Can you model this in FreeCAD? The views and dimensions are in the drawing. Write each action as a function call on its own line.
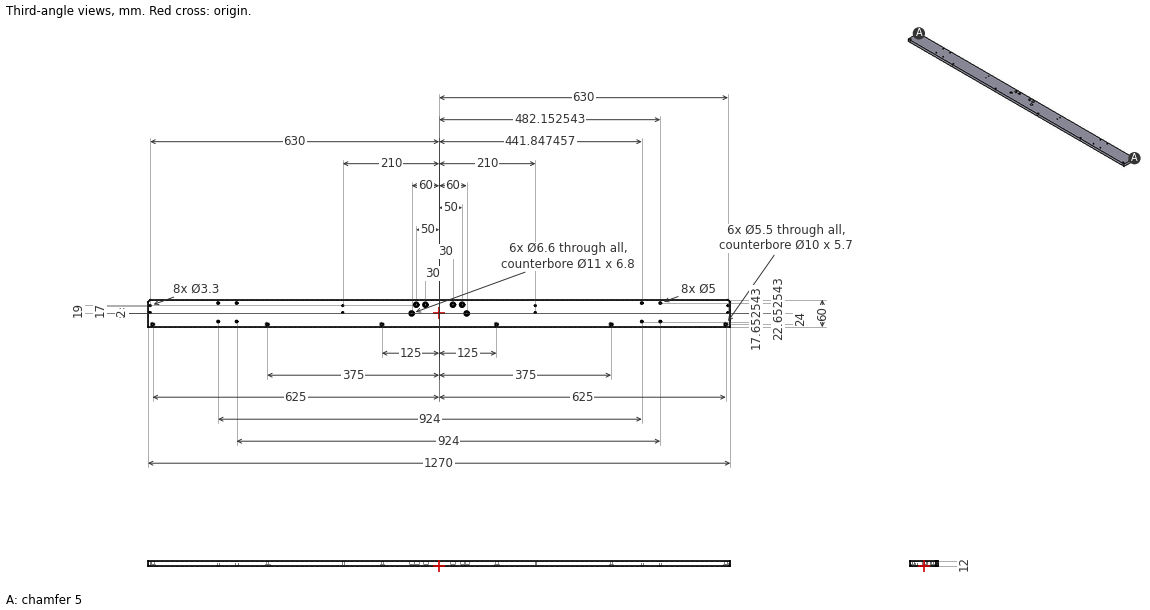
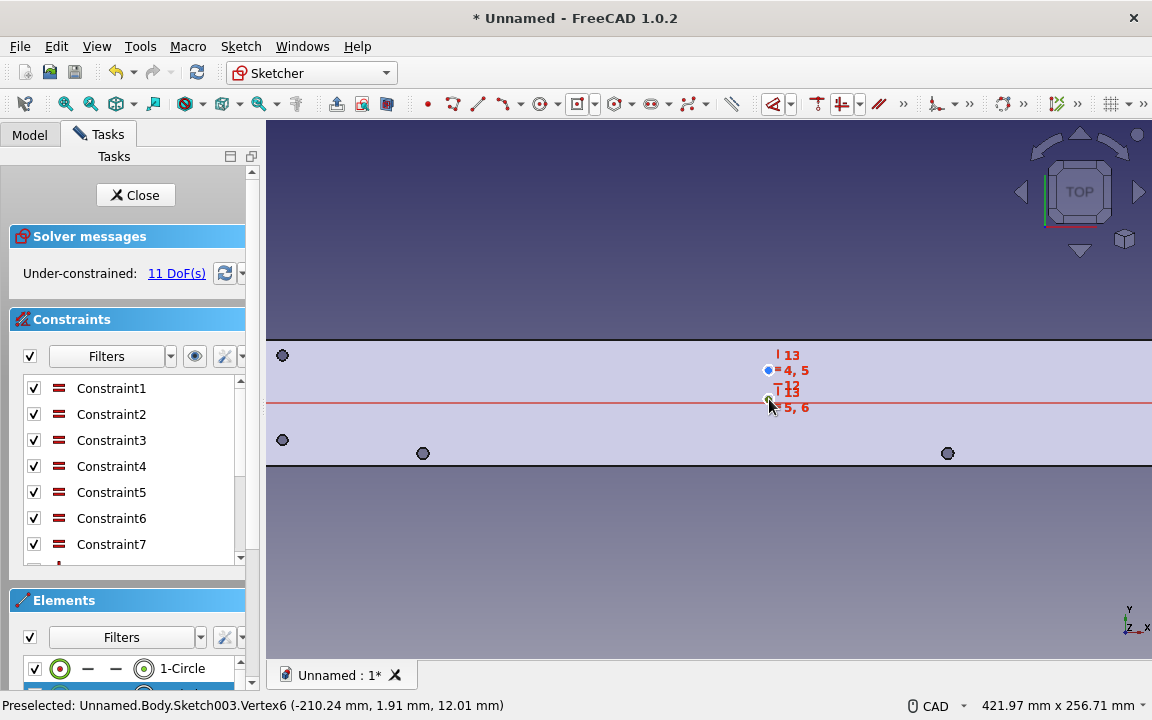
key(h)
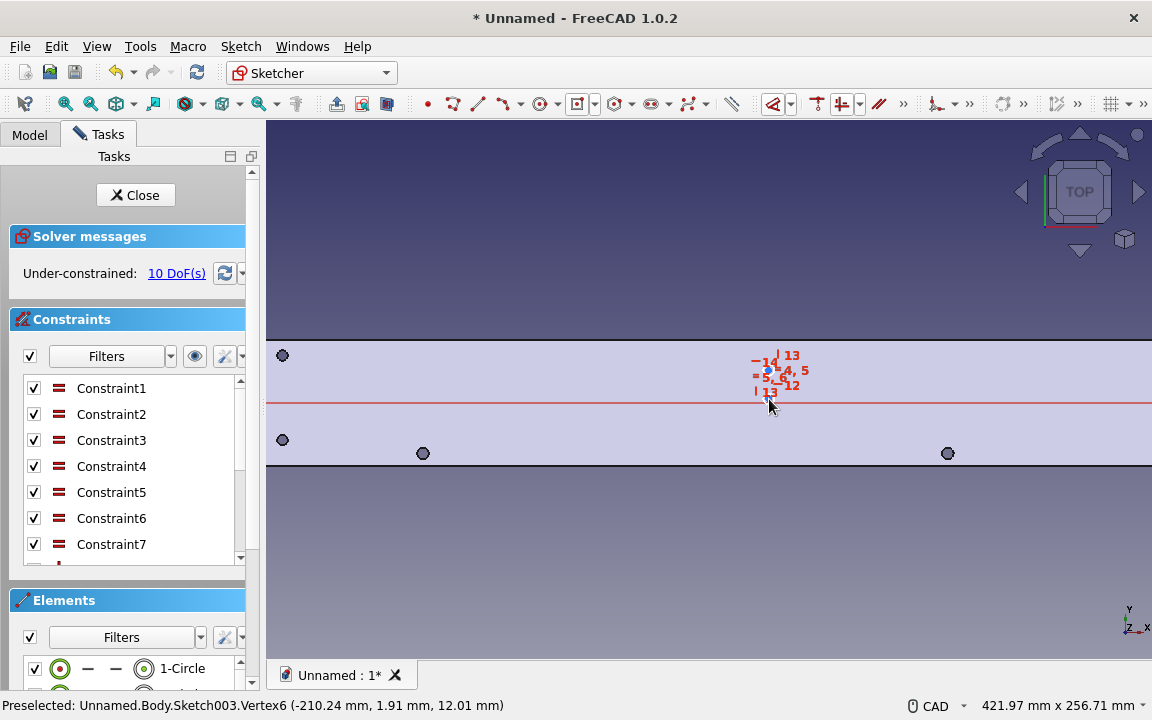
scroll(496, 391, down, 8)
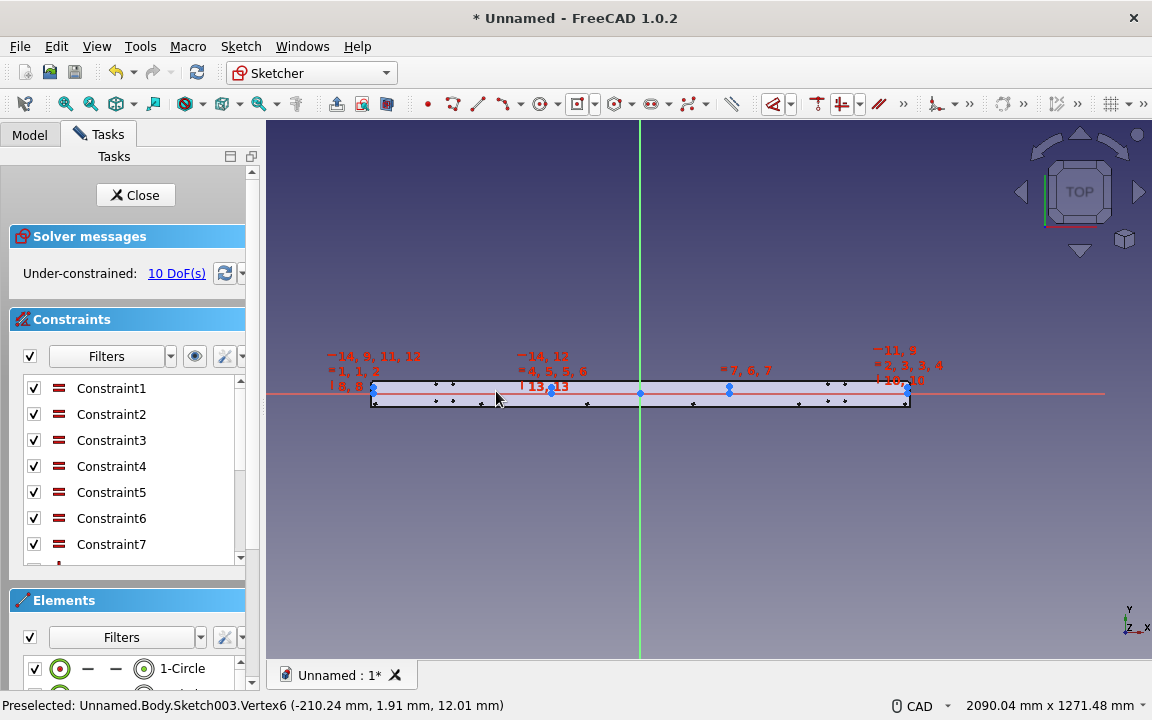
scroll(907, 393, up, 4)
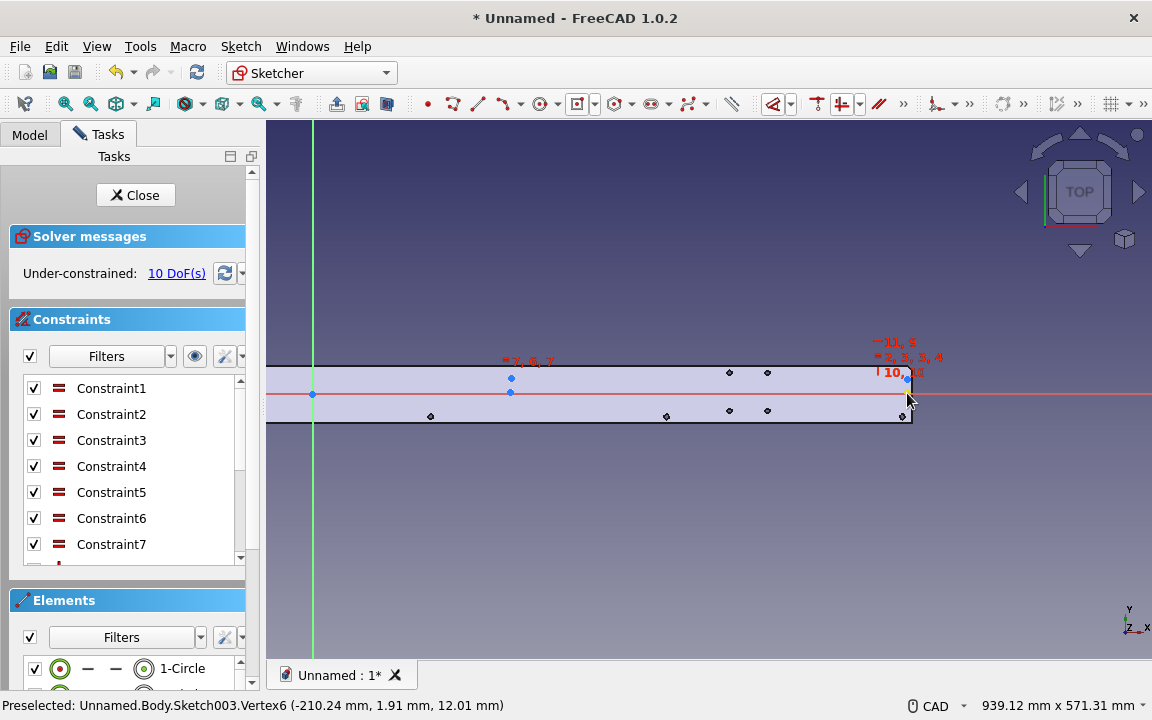
click(907, 392)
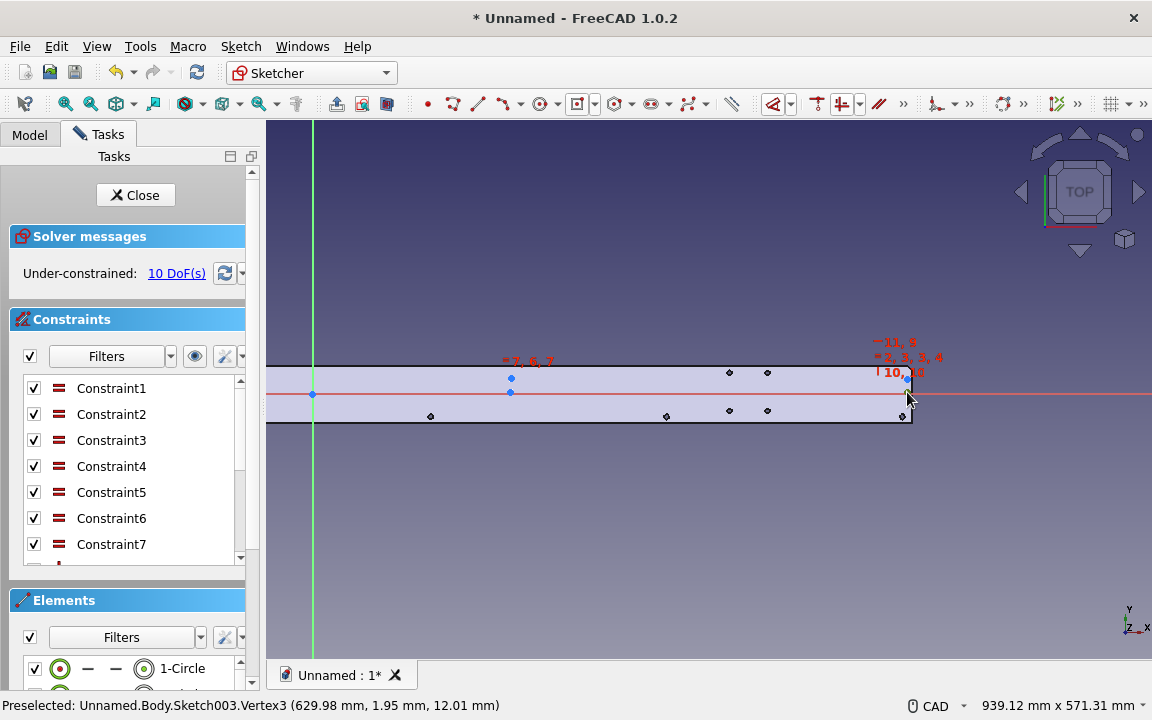
click(511, 392)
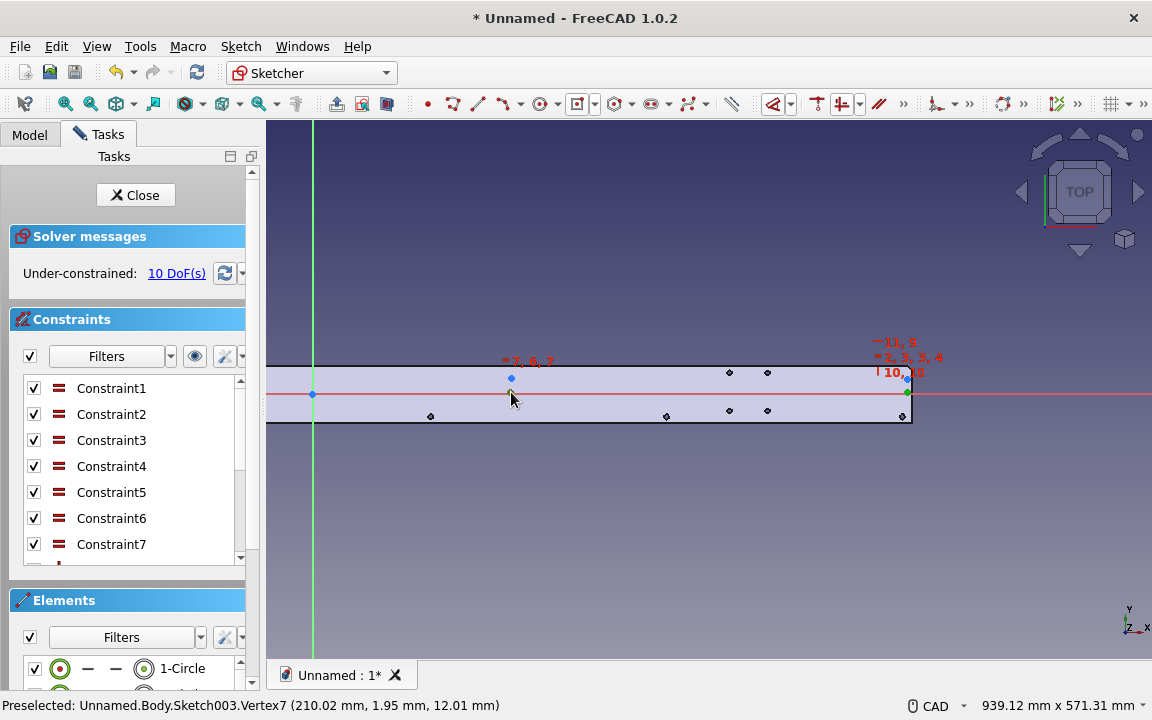
click(860, 104)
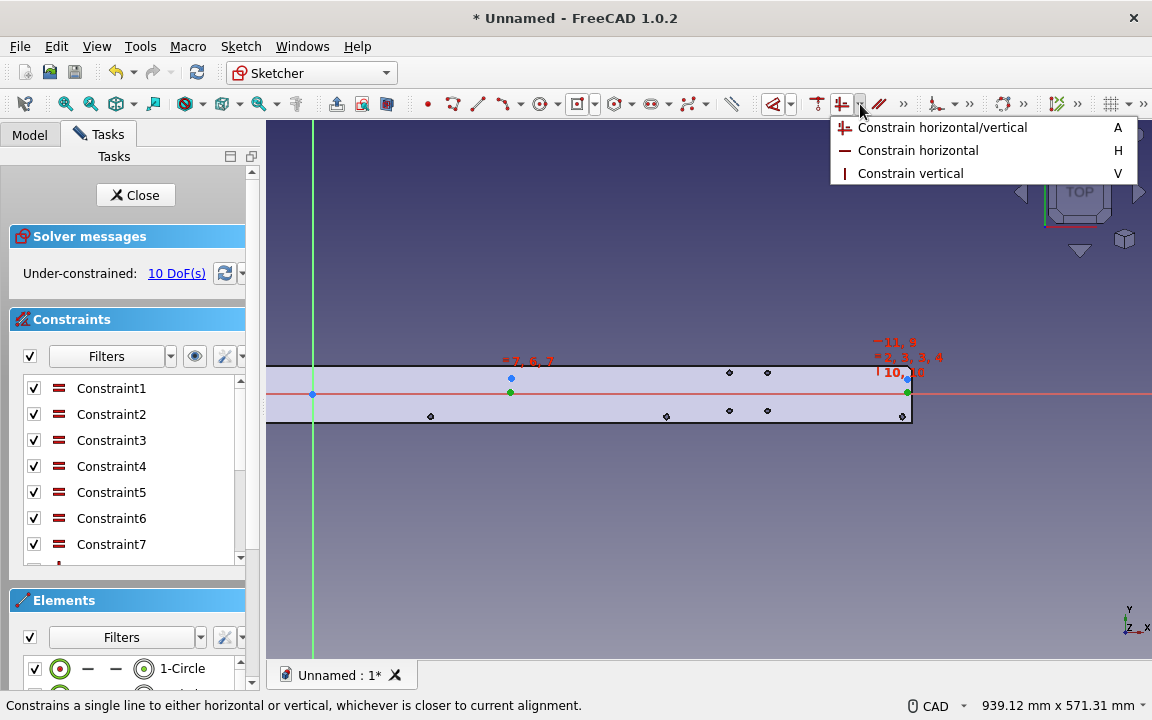
click(984, 150)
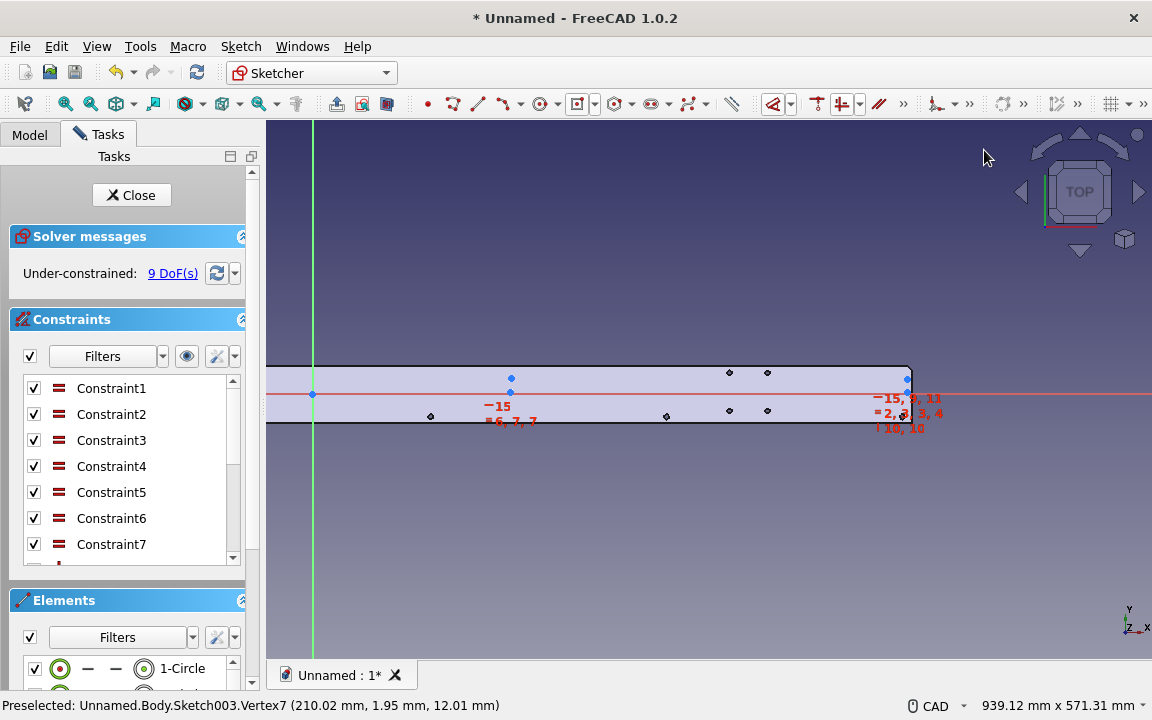
click(511, 392)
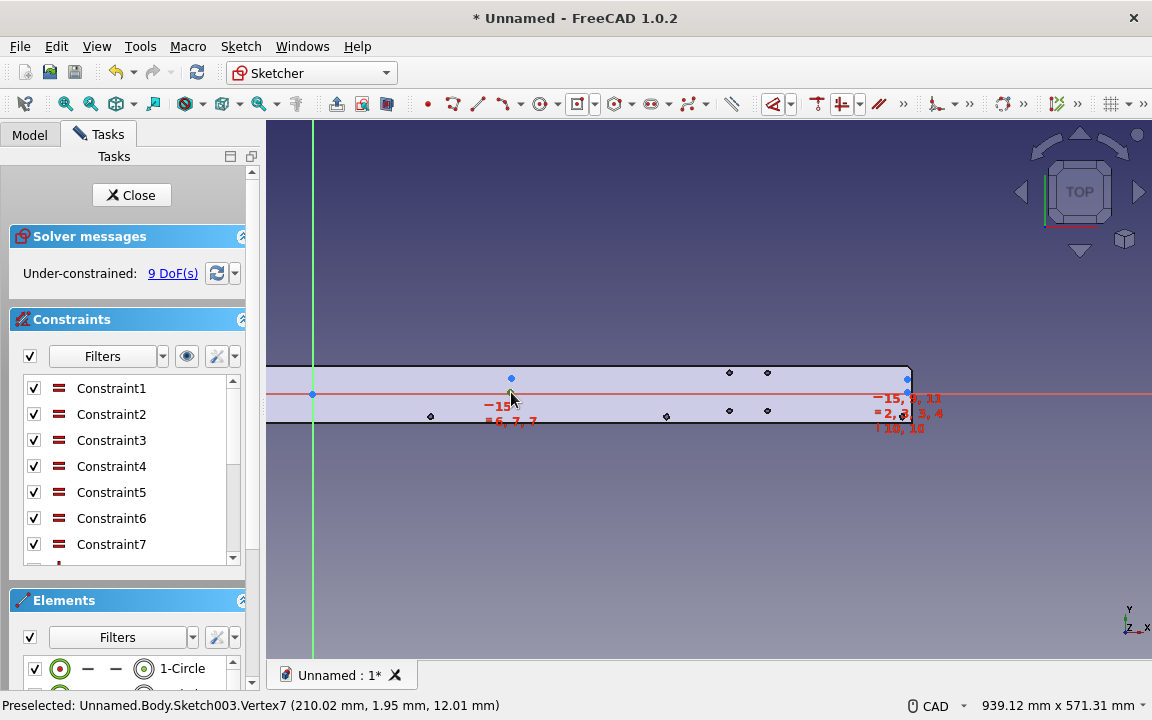
click(511, 379)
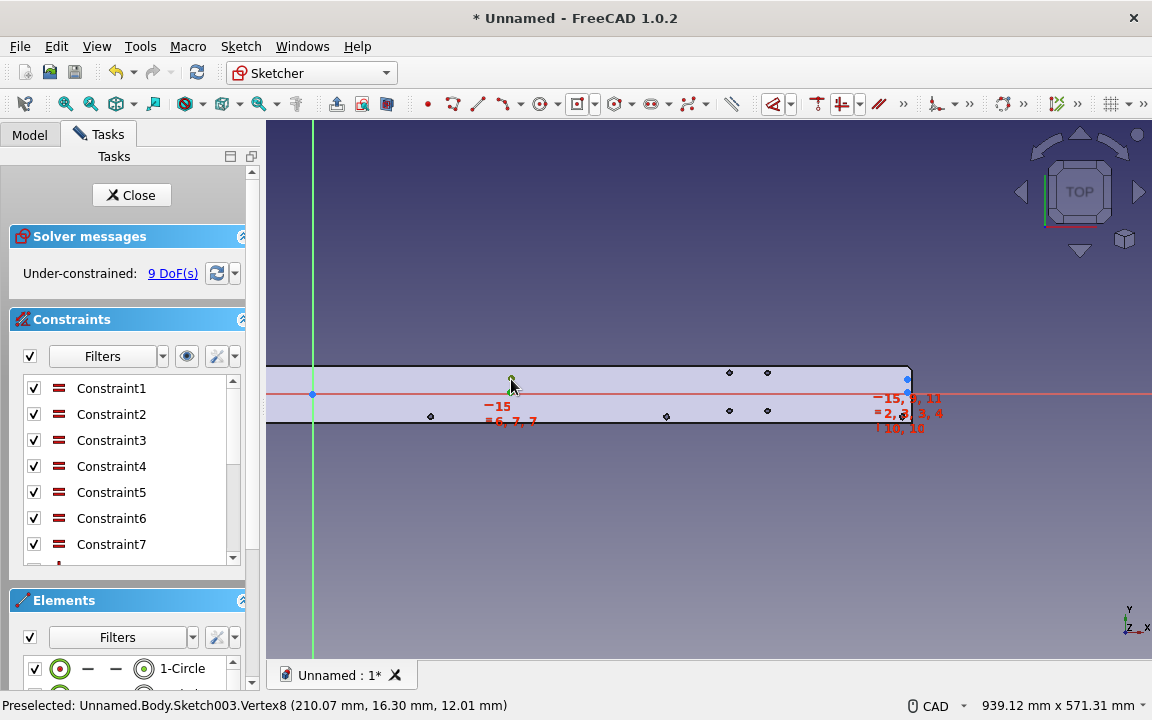
key(v)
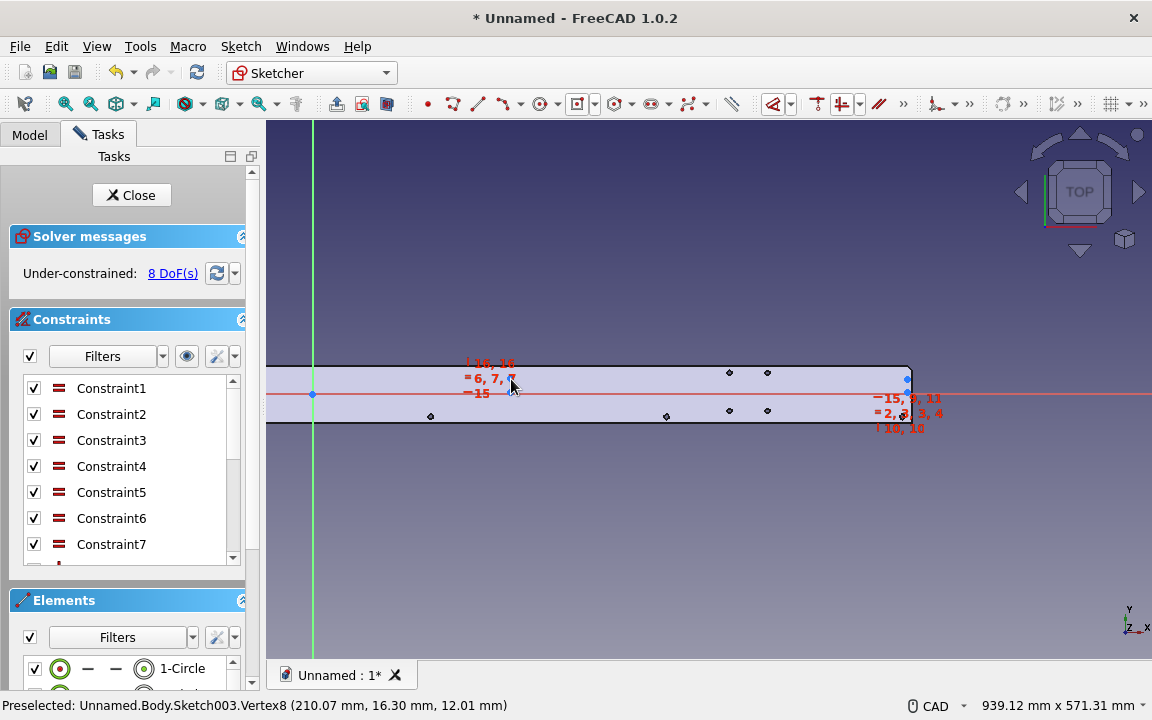
click(907, 379)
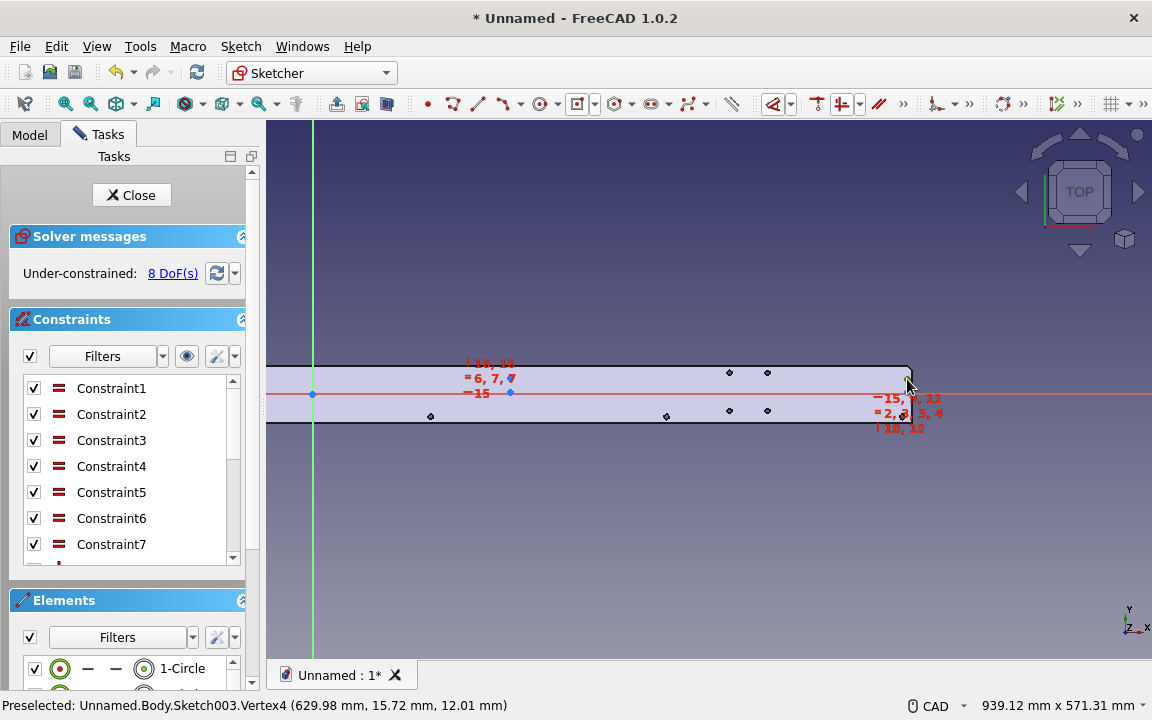
scroll(511, 379, up, 4)